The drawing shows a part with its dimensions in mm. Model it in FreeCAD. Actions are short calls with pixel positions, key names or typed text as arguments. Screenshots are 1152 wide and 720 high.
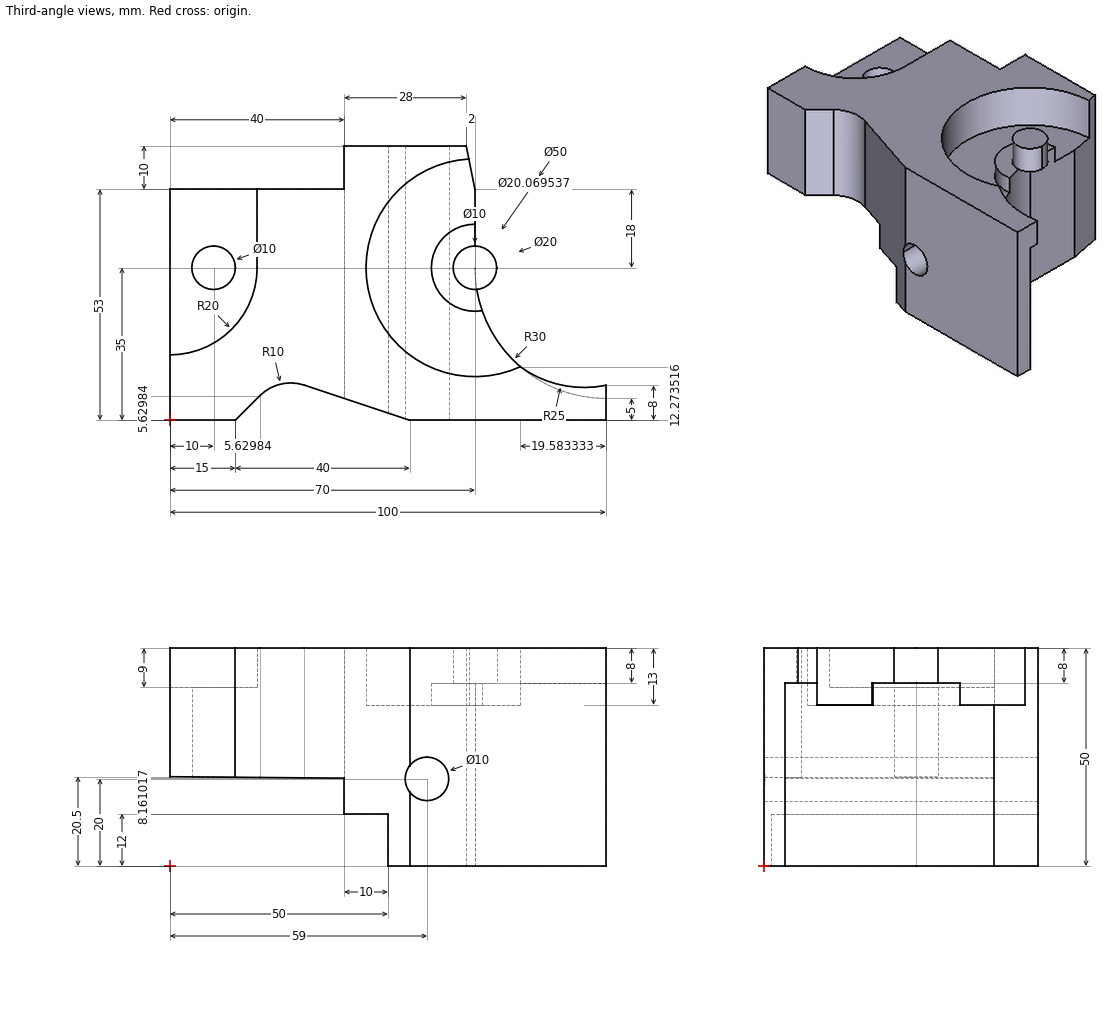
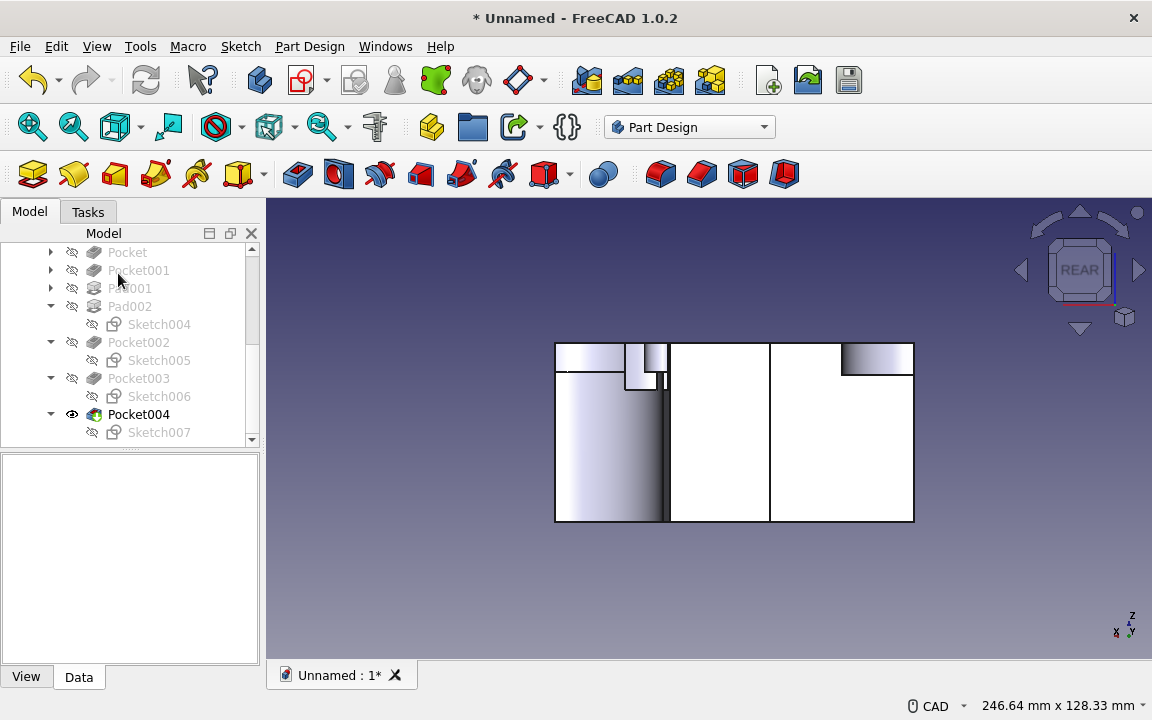
key(v)
key(f)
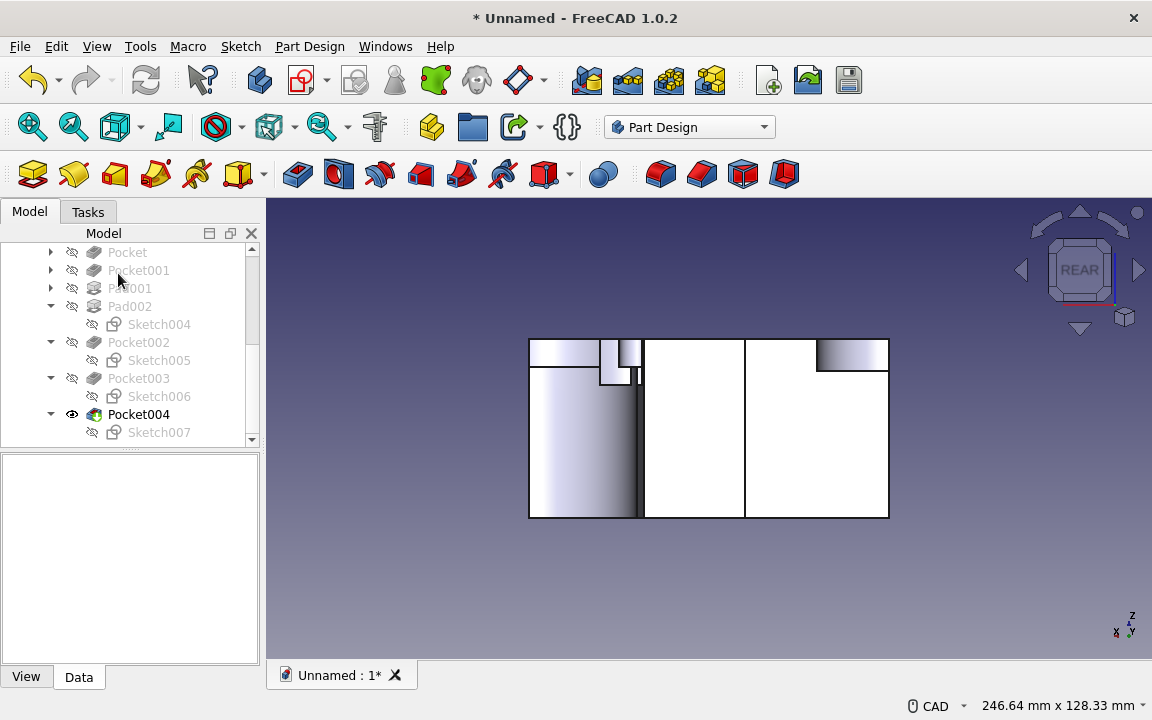
click(695, 402)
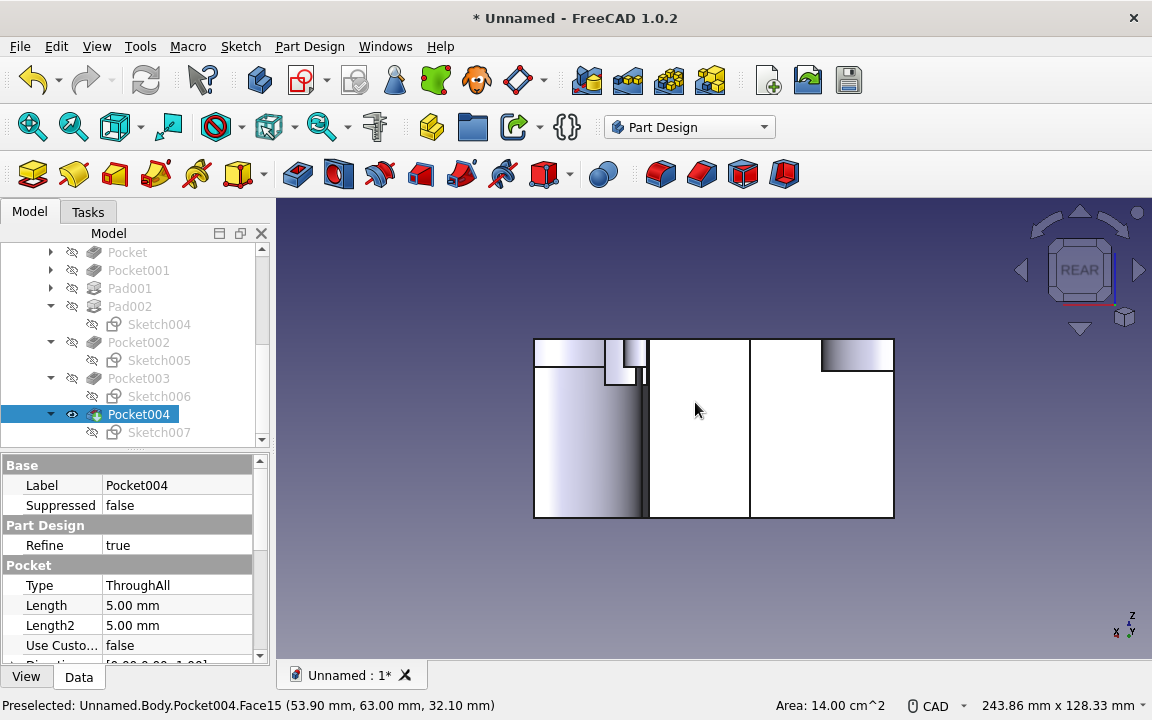
click(300, 80)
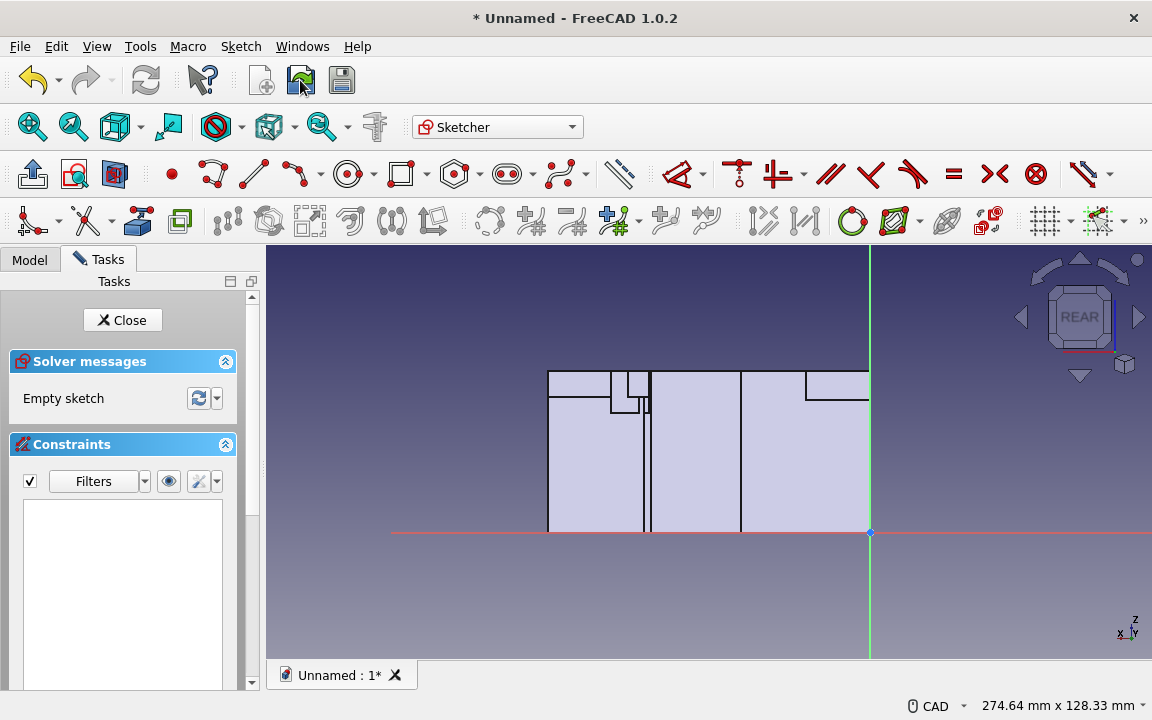
scroll(686, 471, up, 10)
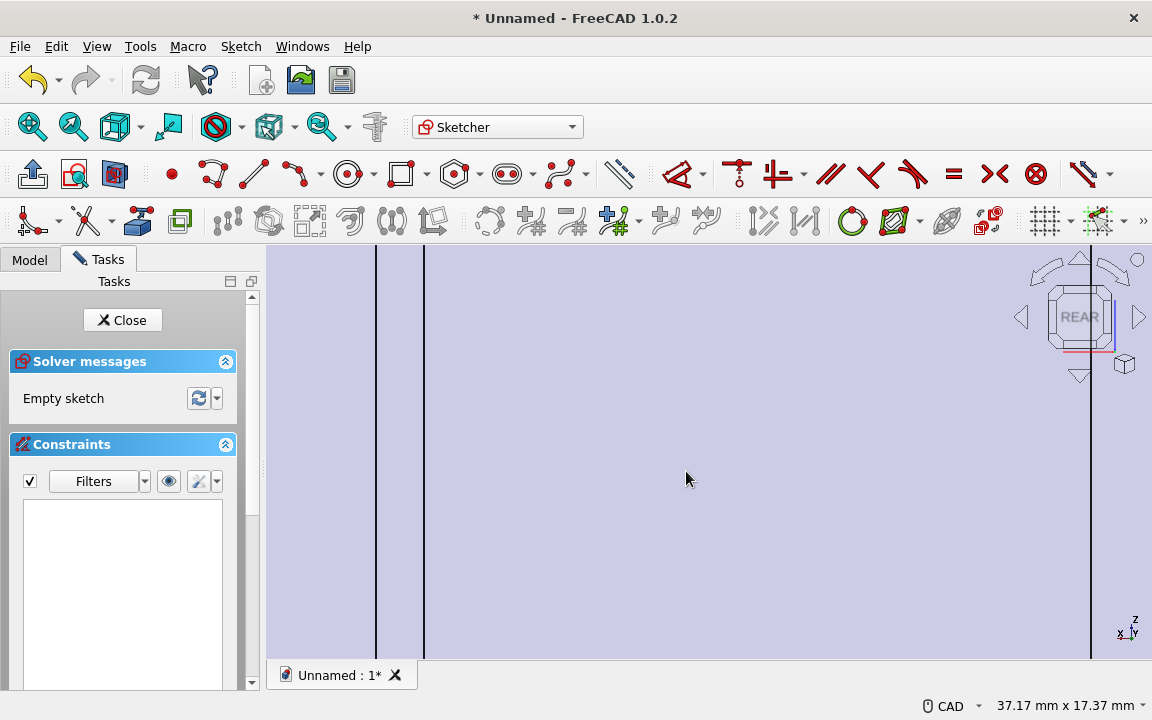
key(g)
key(c)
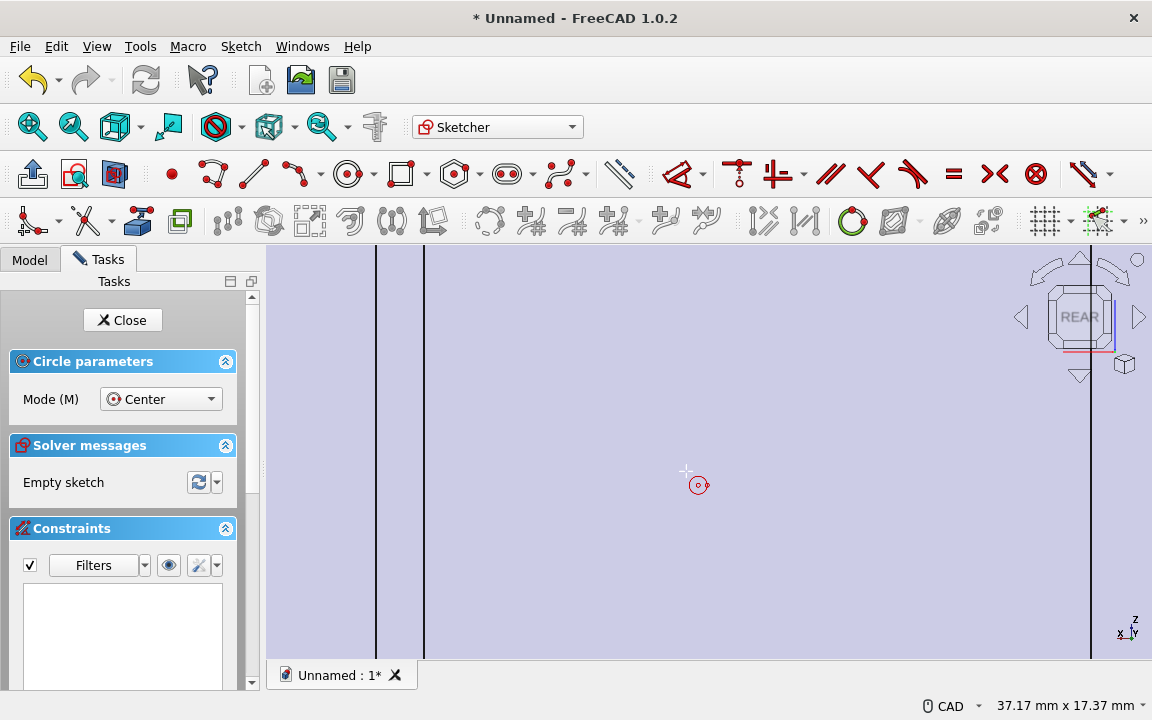
click(638, 446)
click(723, 362)
key(Escape)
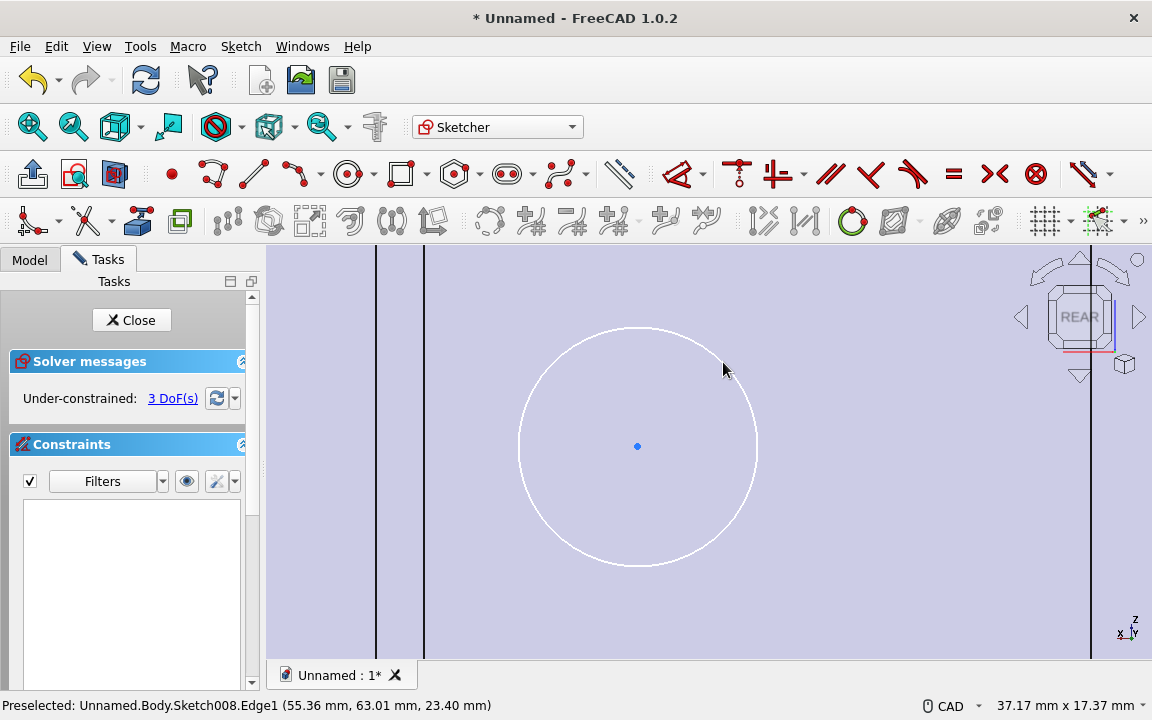
click(676, 174)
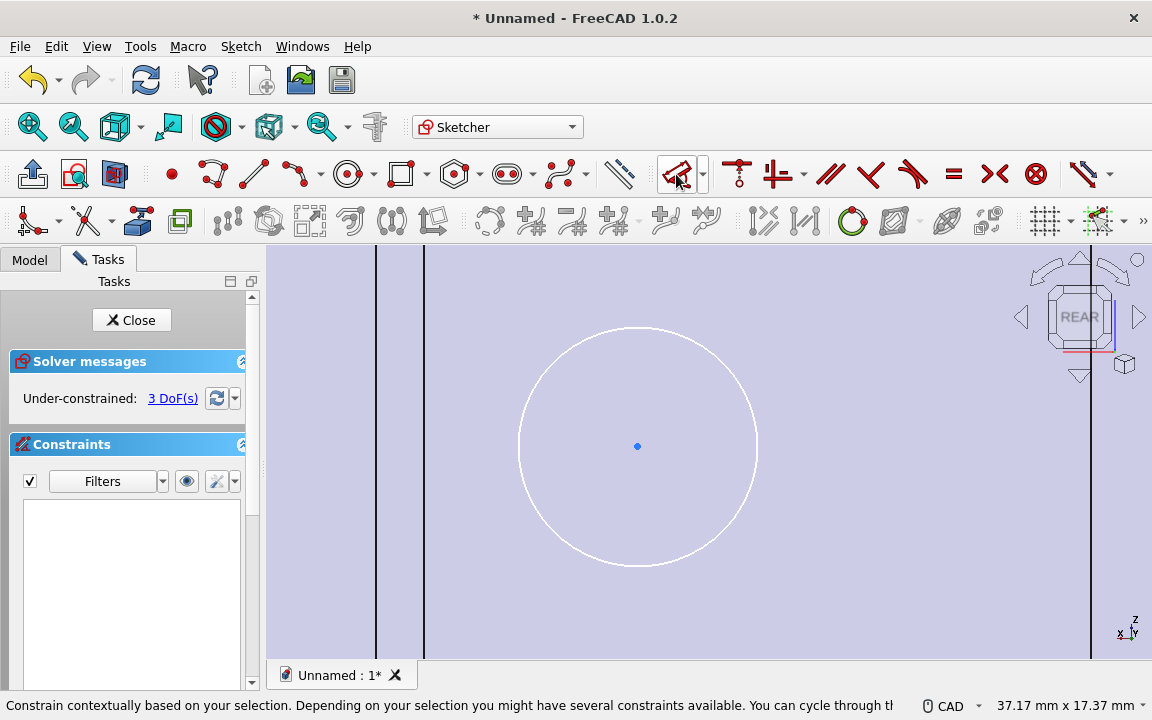
click(722, 362)
click(744, 339)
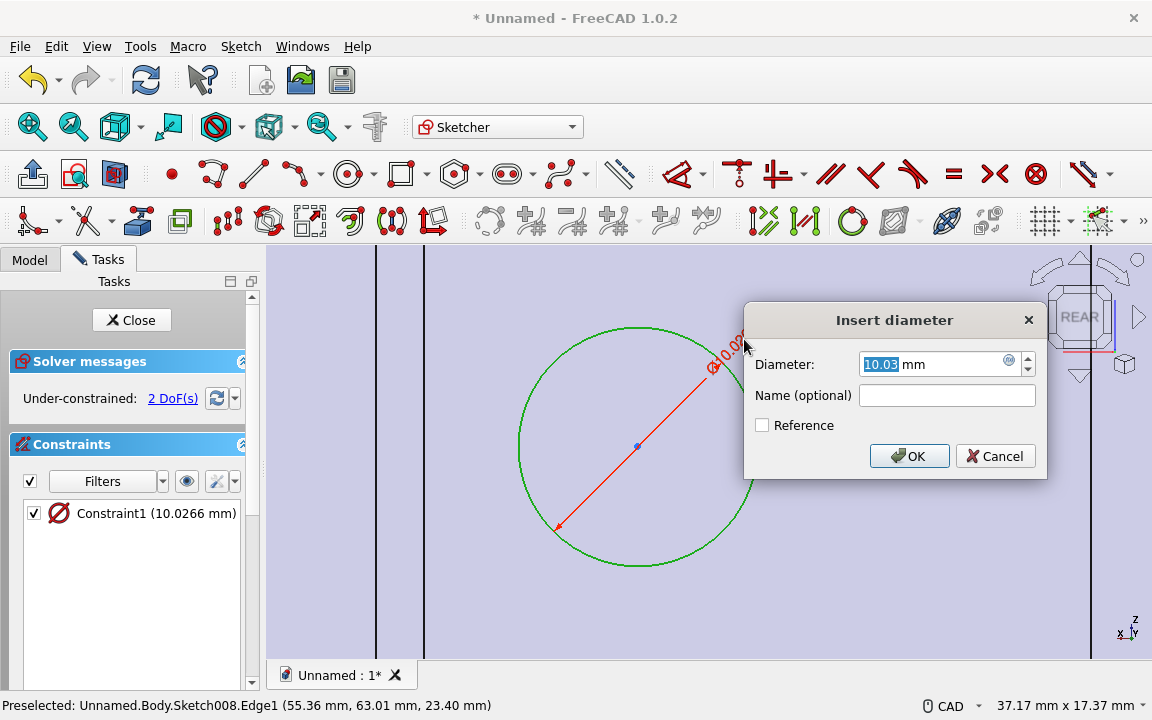
text(10)
key(Return)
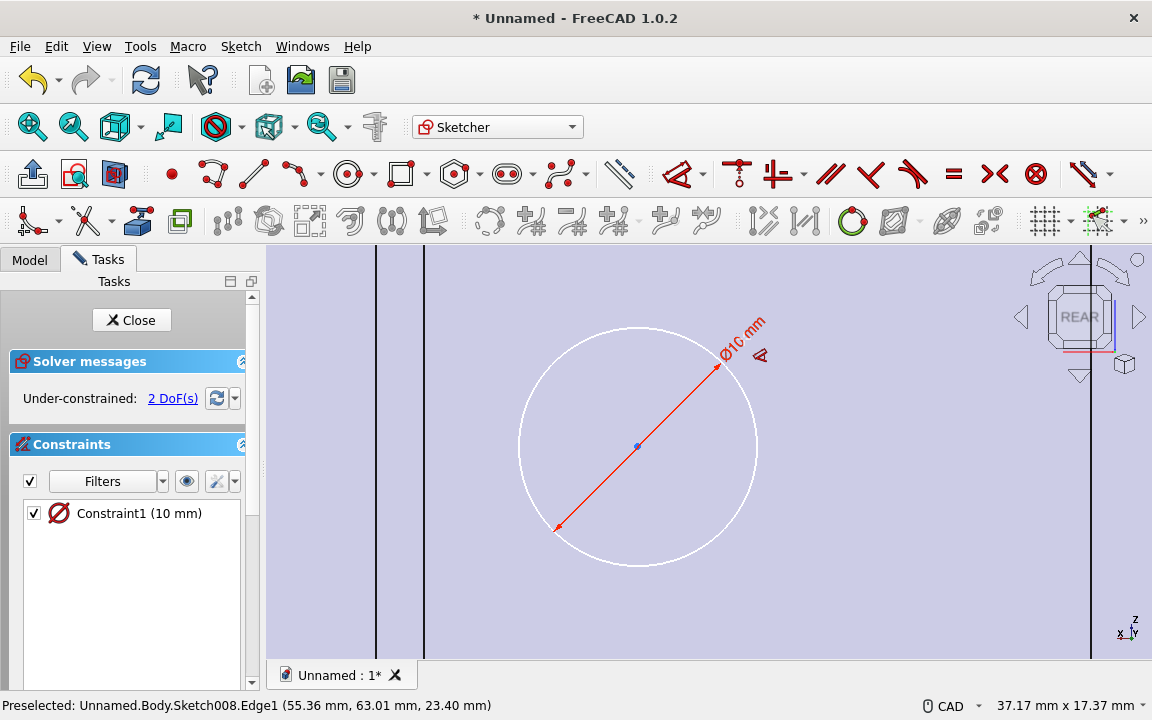
click(638, 447)
click(813, 413)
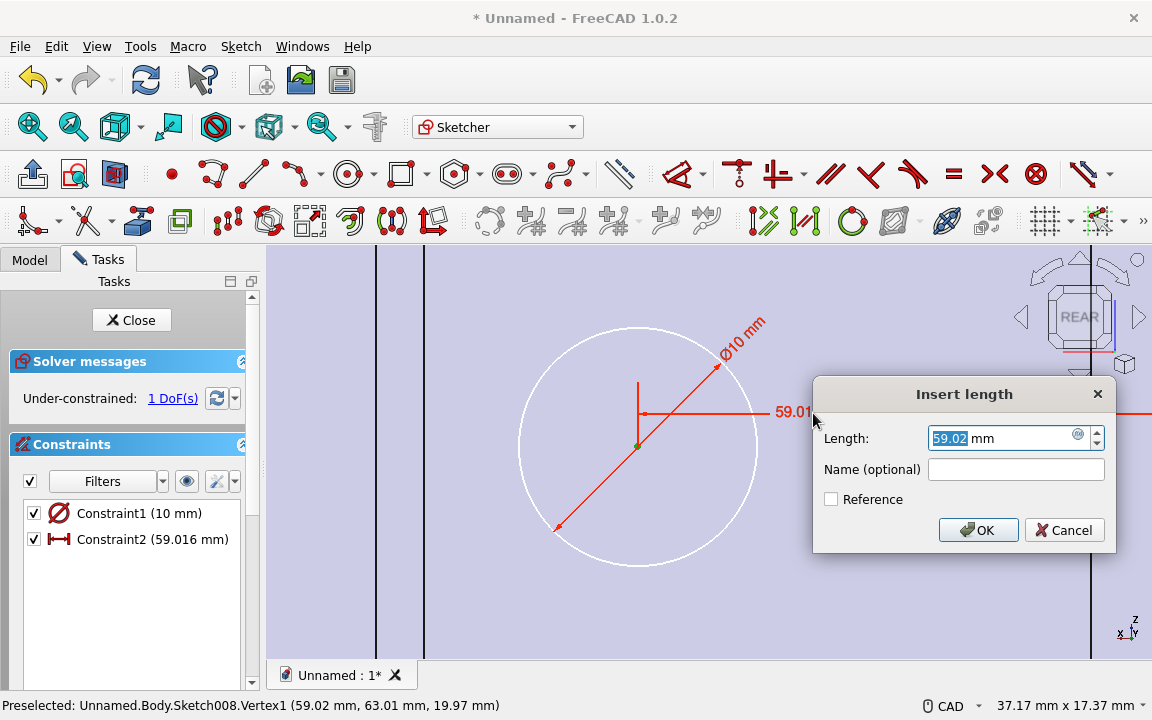
text(59)
key(Return)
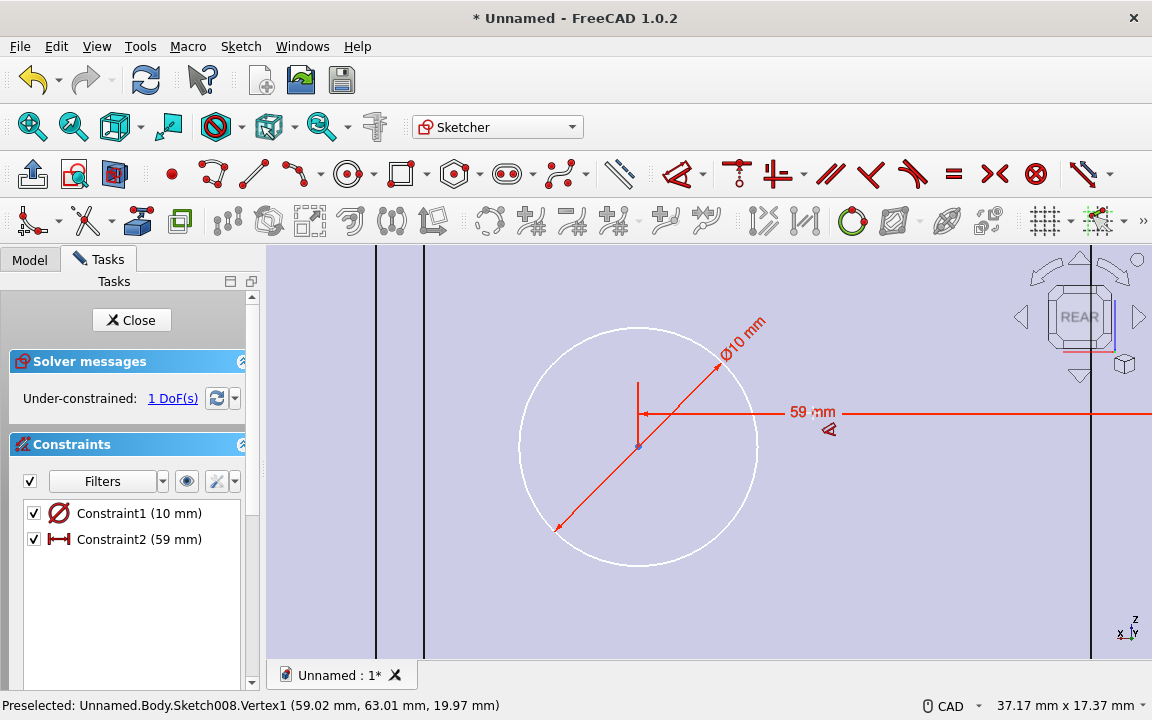
click(638, 447)
click(604, 539)